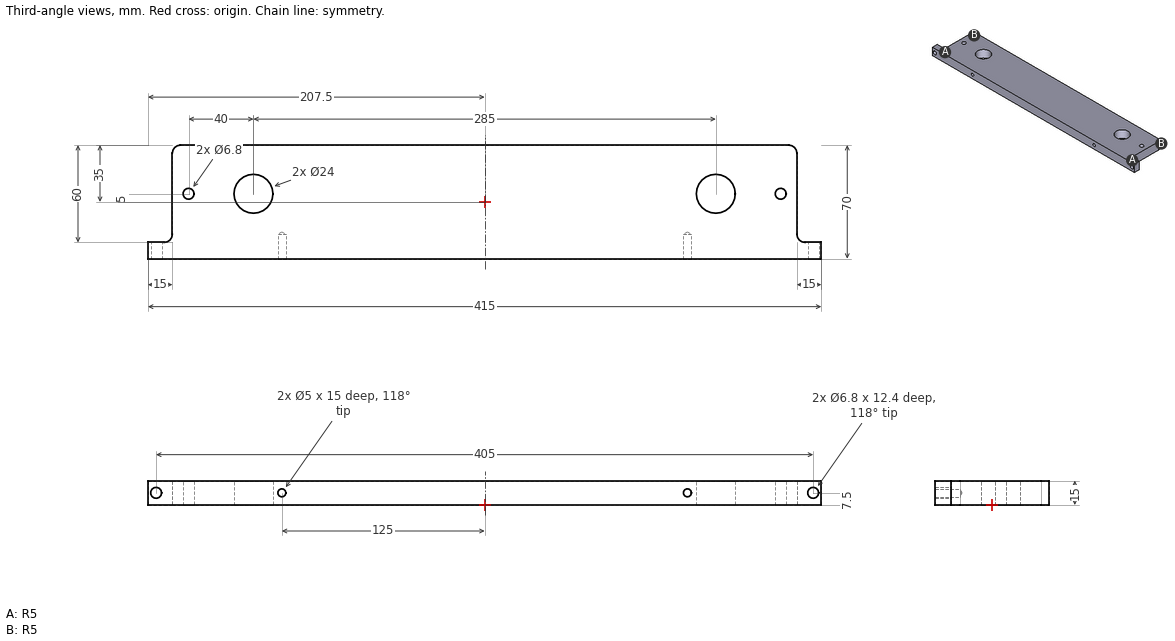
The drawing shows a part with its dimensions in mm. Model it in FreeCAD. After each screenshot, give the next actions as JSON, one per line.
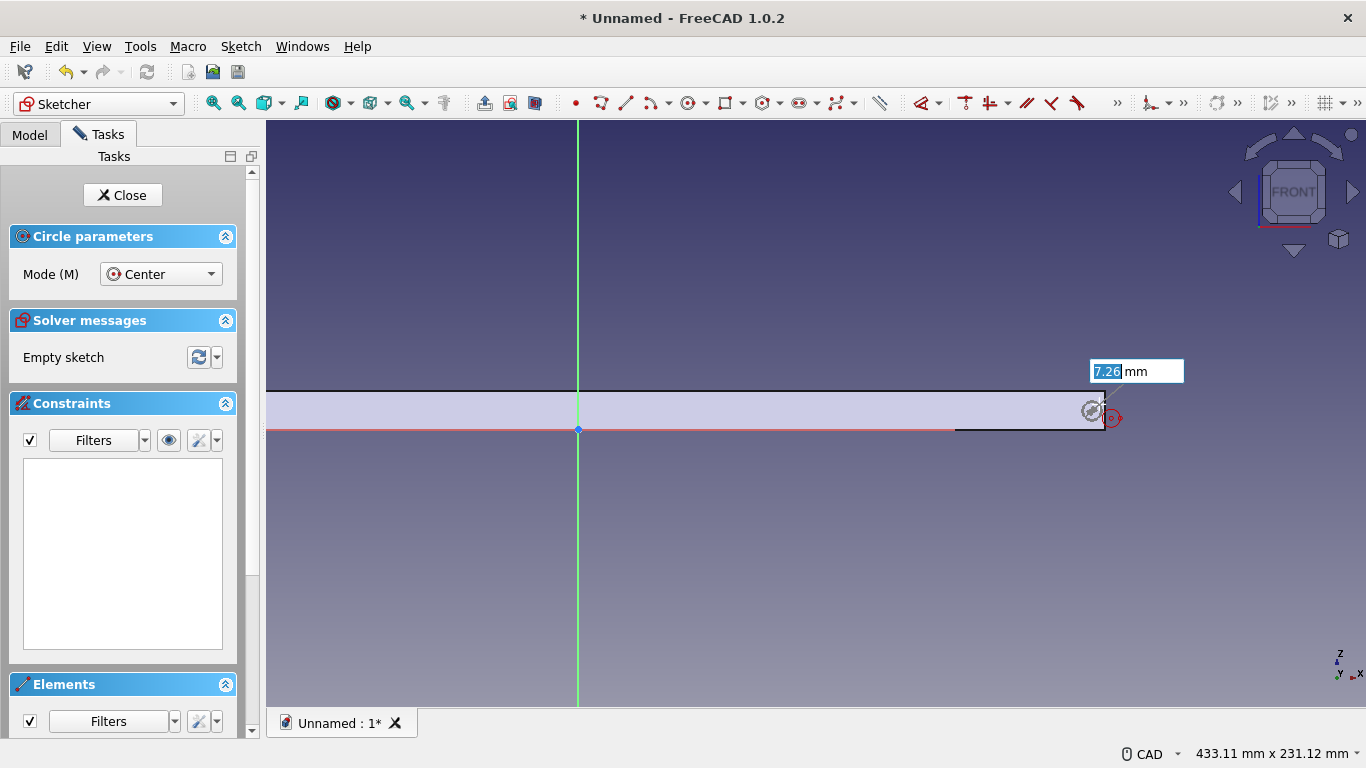
{"action": "type", "text": "6.8"}
{"action": "key", "text": "Return"}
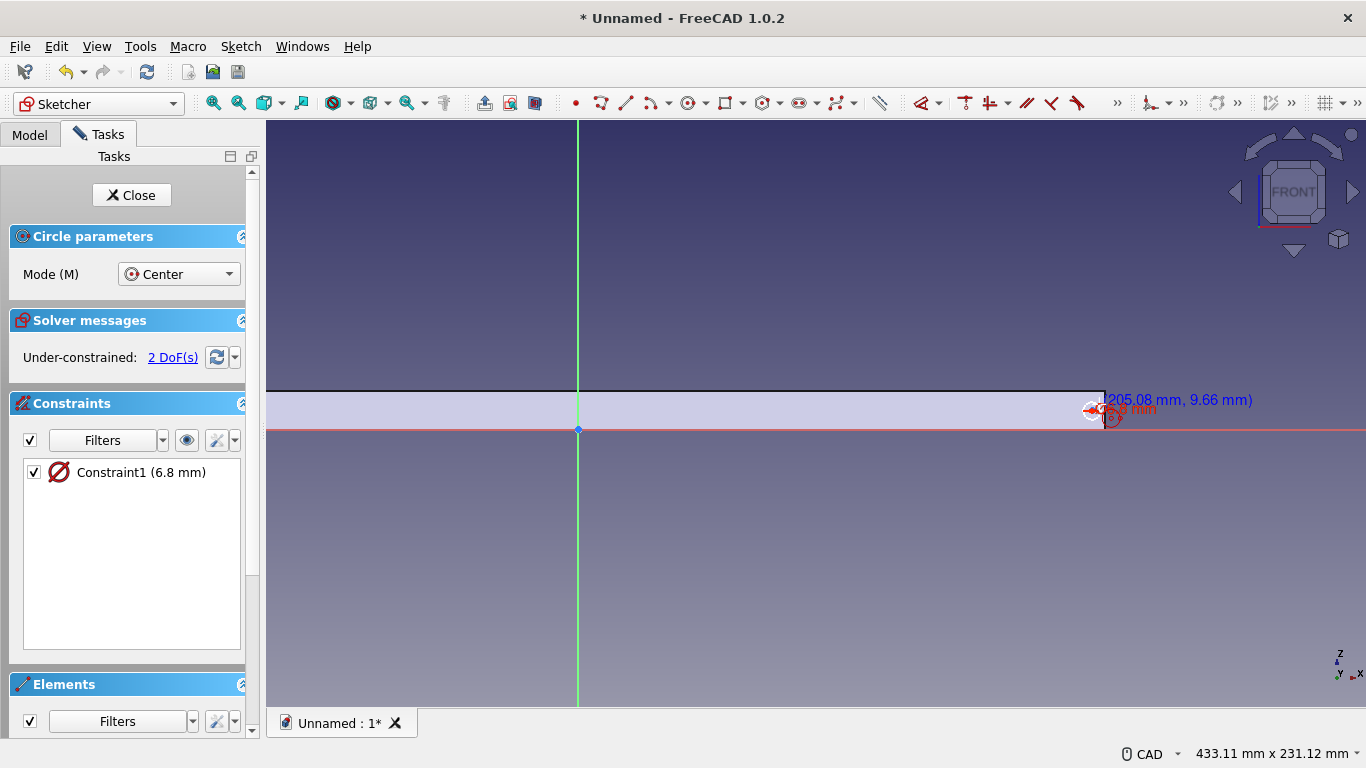
{"action": "scroll", "coordinate": [1092, 409], "scroll_direction": "down", "scroll_amount": 2}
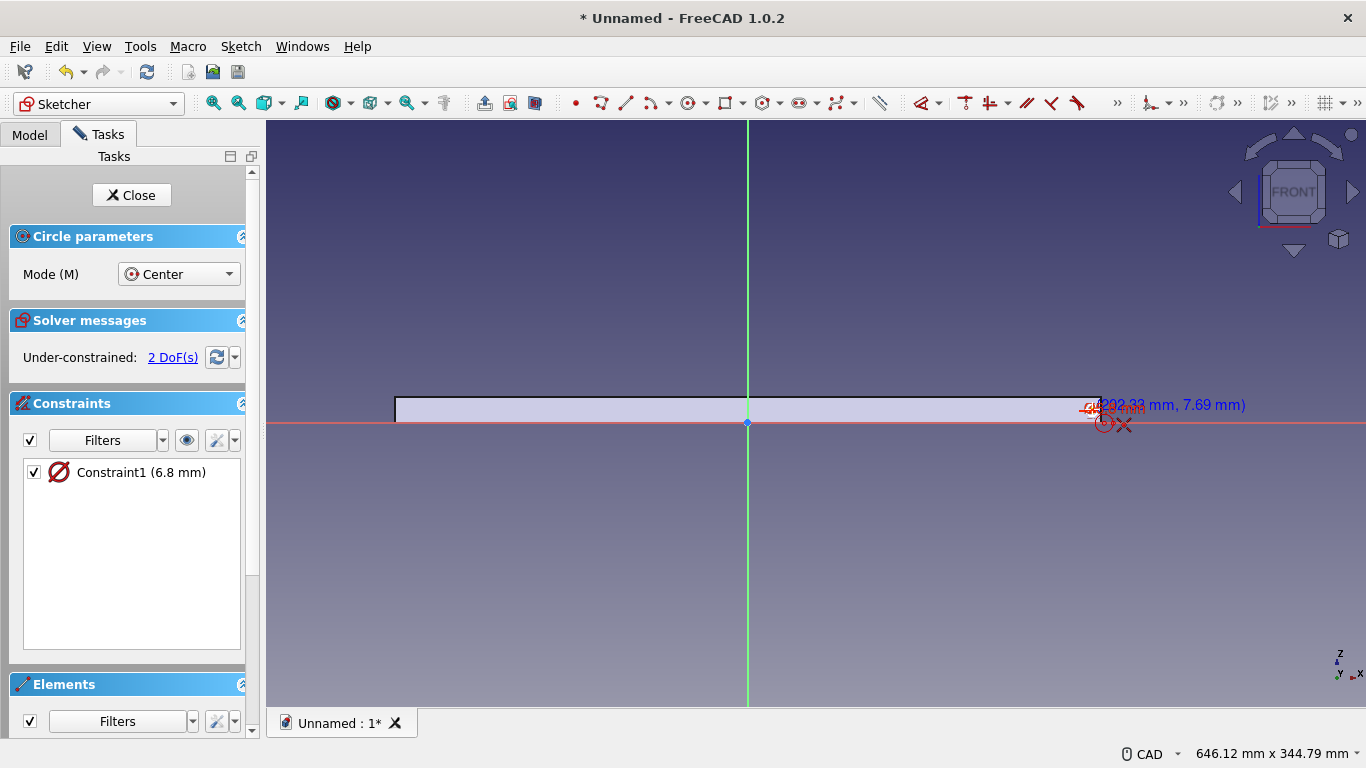
{"action": "scroll", "coordinate": [403, 410], "scroll_direction": "up", "scroll_amount": 7}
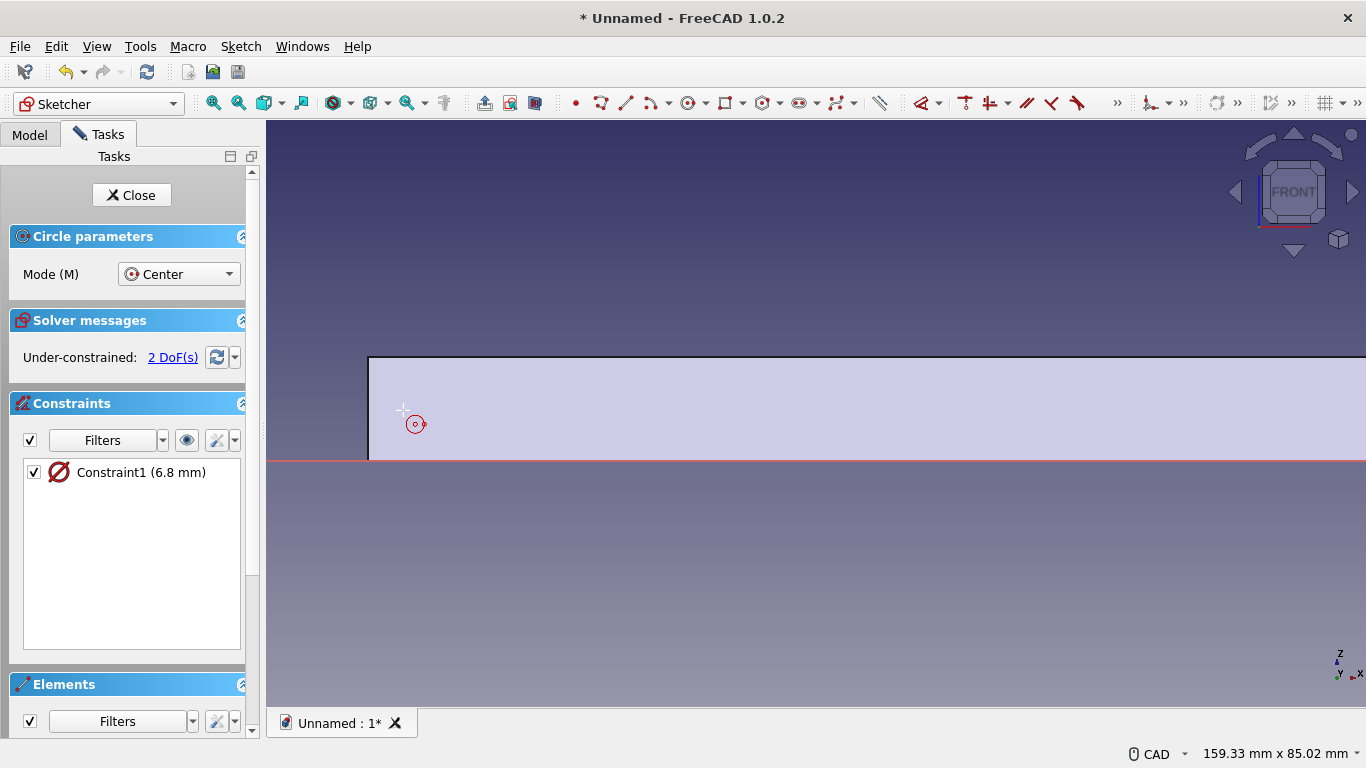
{"action": "scroll", "coordinate": [403, 410], "scroll_direction": "down", "scroll_amount": 7}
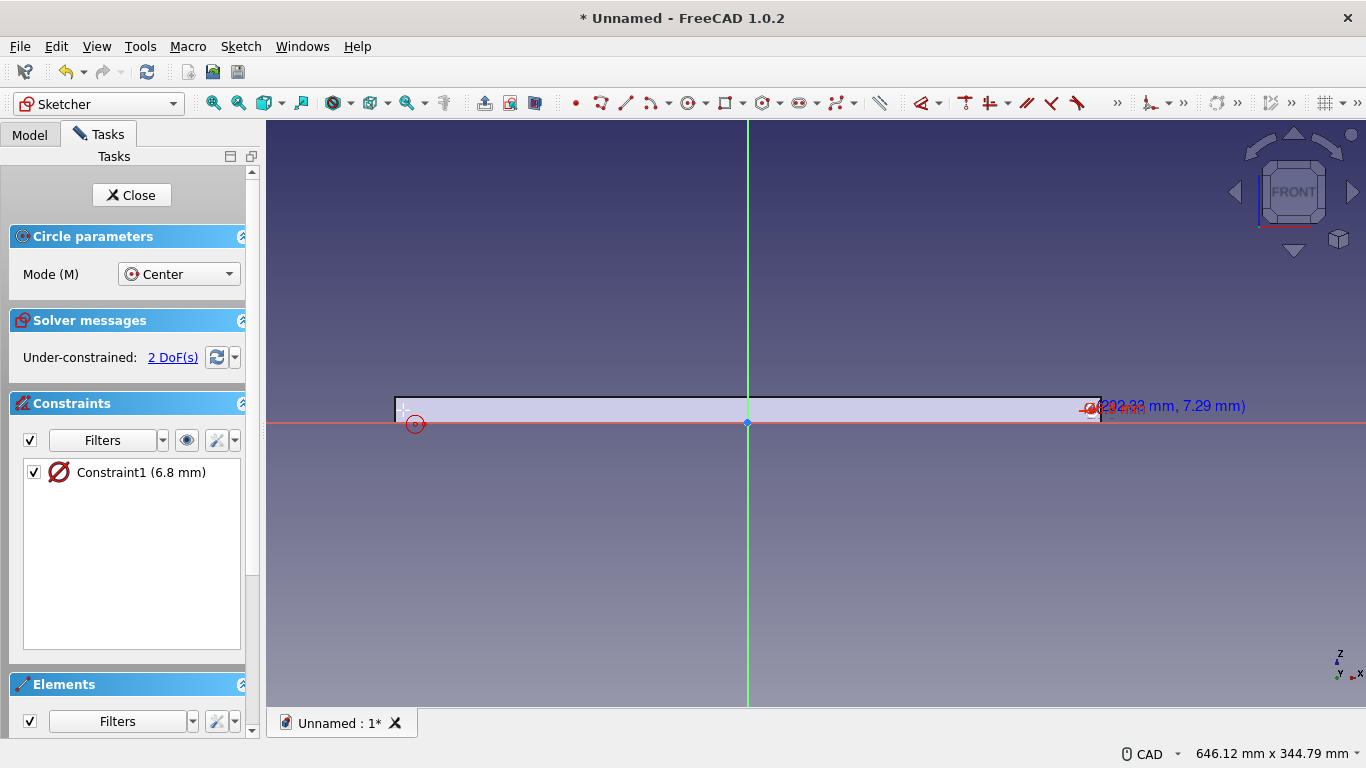
{"action": "scroll", "coordinate": [403, 410], "scroll_direction": "up", "scroll_amount": 2}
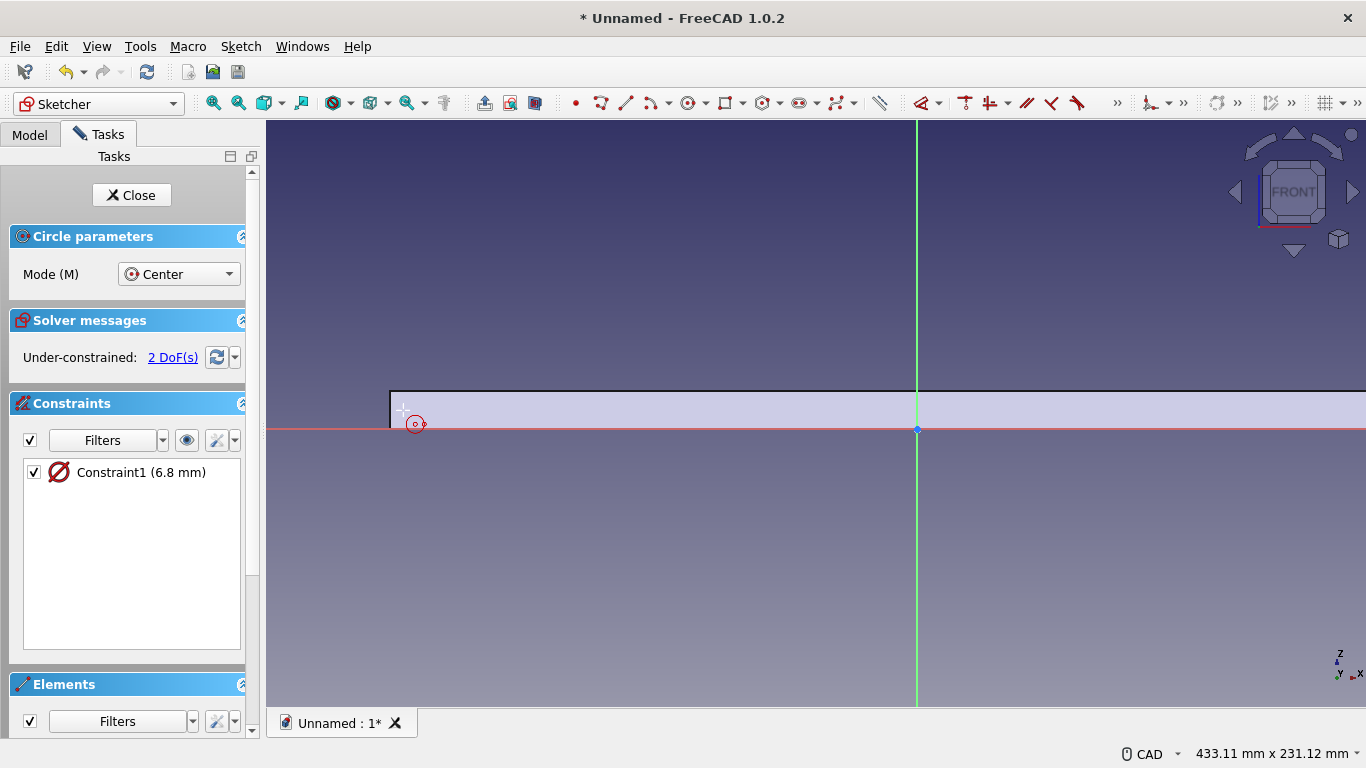
{"action": "left_click", "coordinate": [403, 410]}
{"action": "mouse_move", "coordinate": [409, 404]}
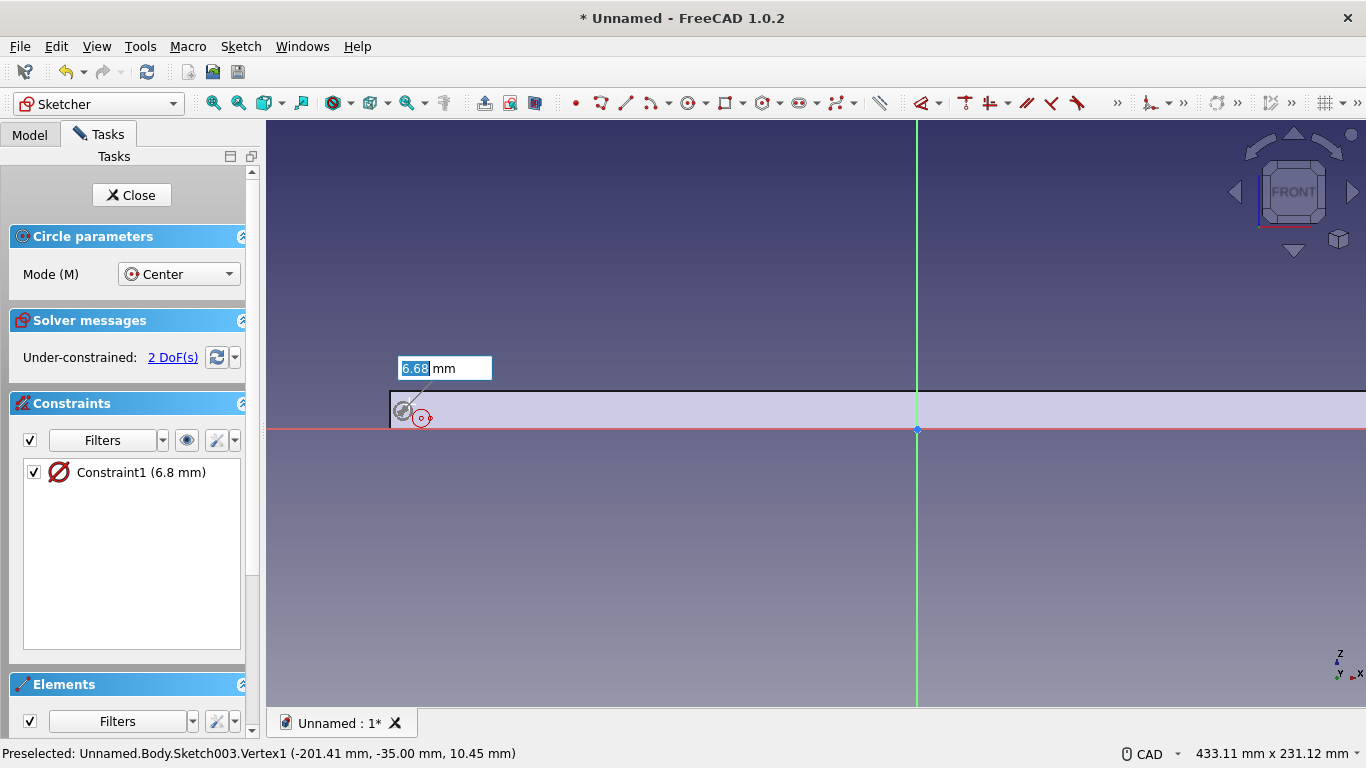
{"action": "type", "text": "6.8"}
{"action": "key", "text": "Return"}
{"action": "key", "text": "Escape"}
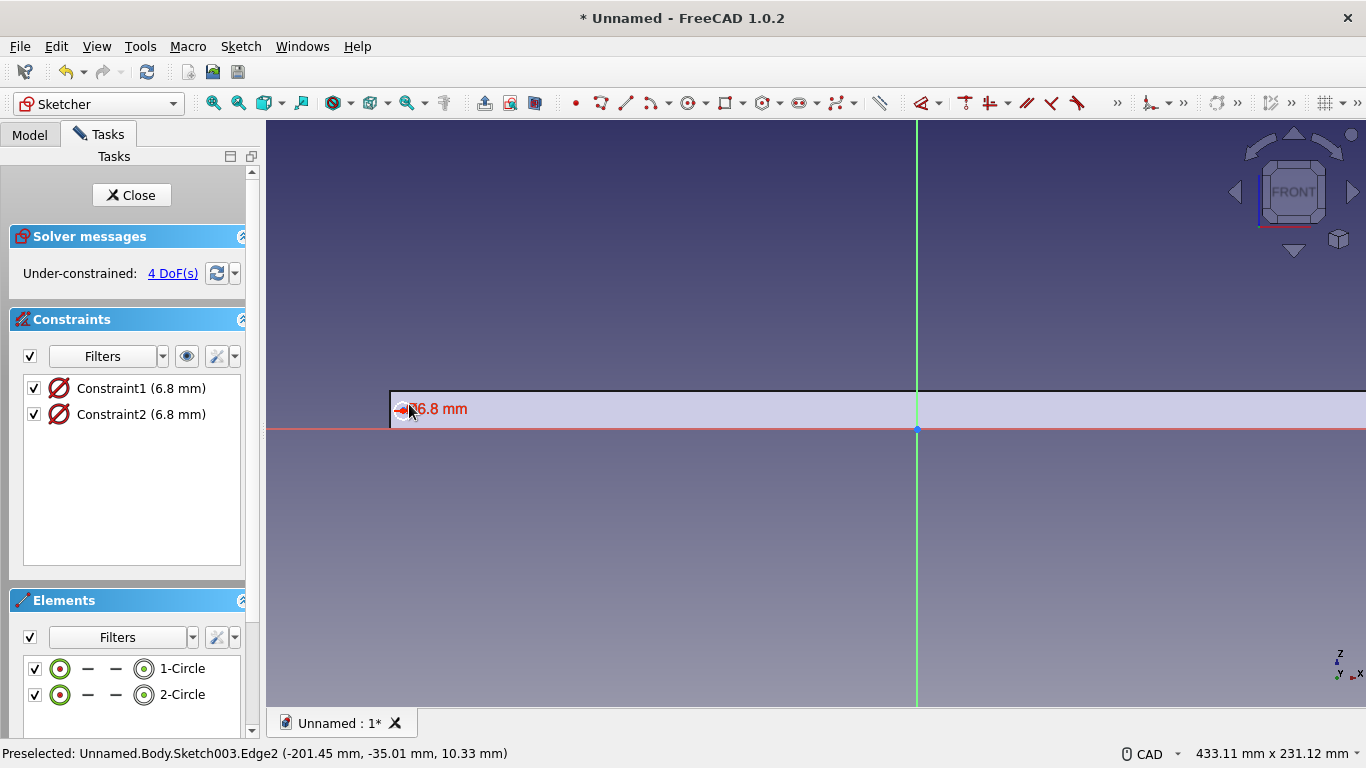
{"action": "scroll", "coordinate": [402, 410], "scroll_direction": "down", "scroll_amount": 2}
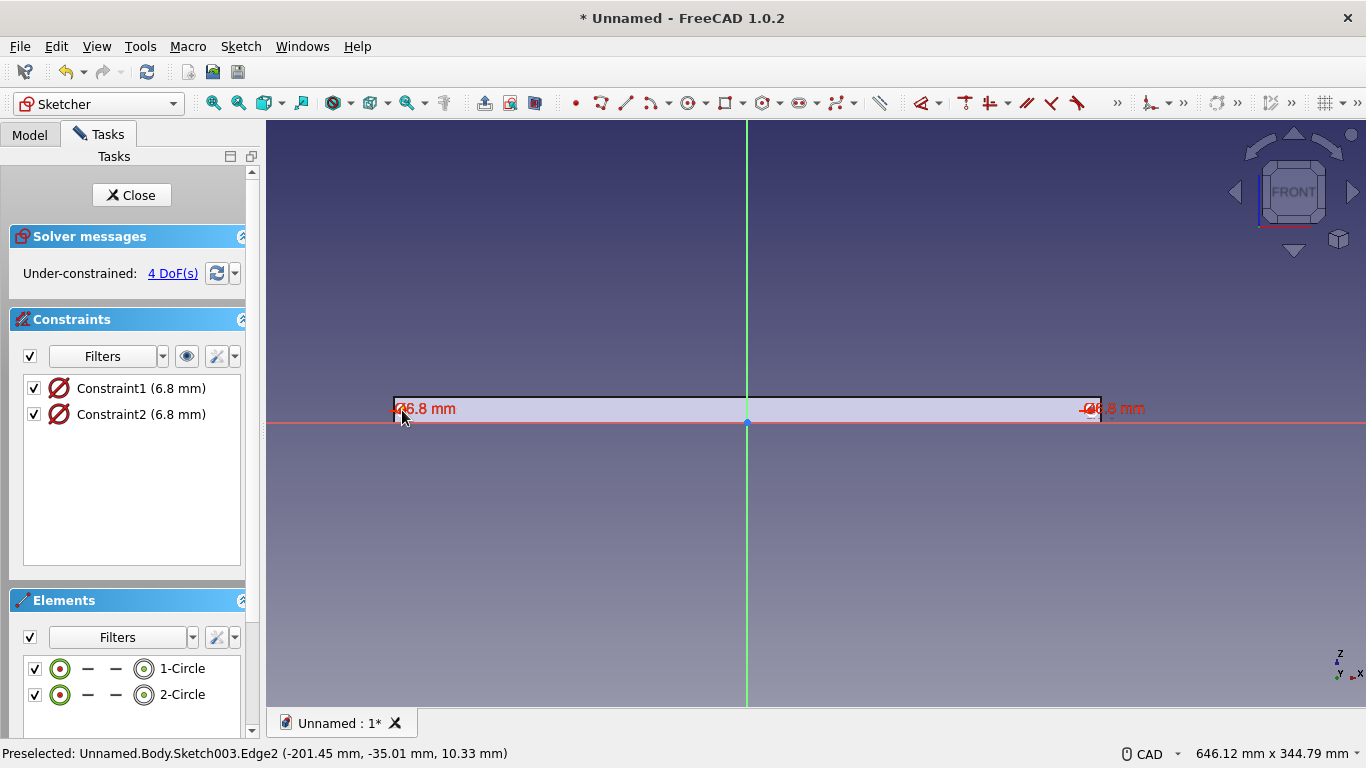
{"action": "left_click", "coordinate": [1092, 411]}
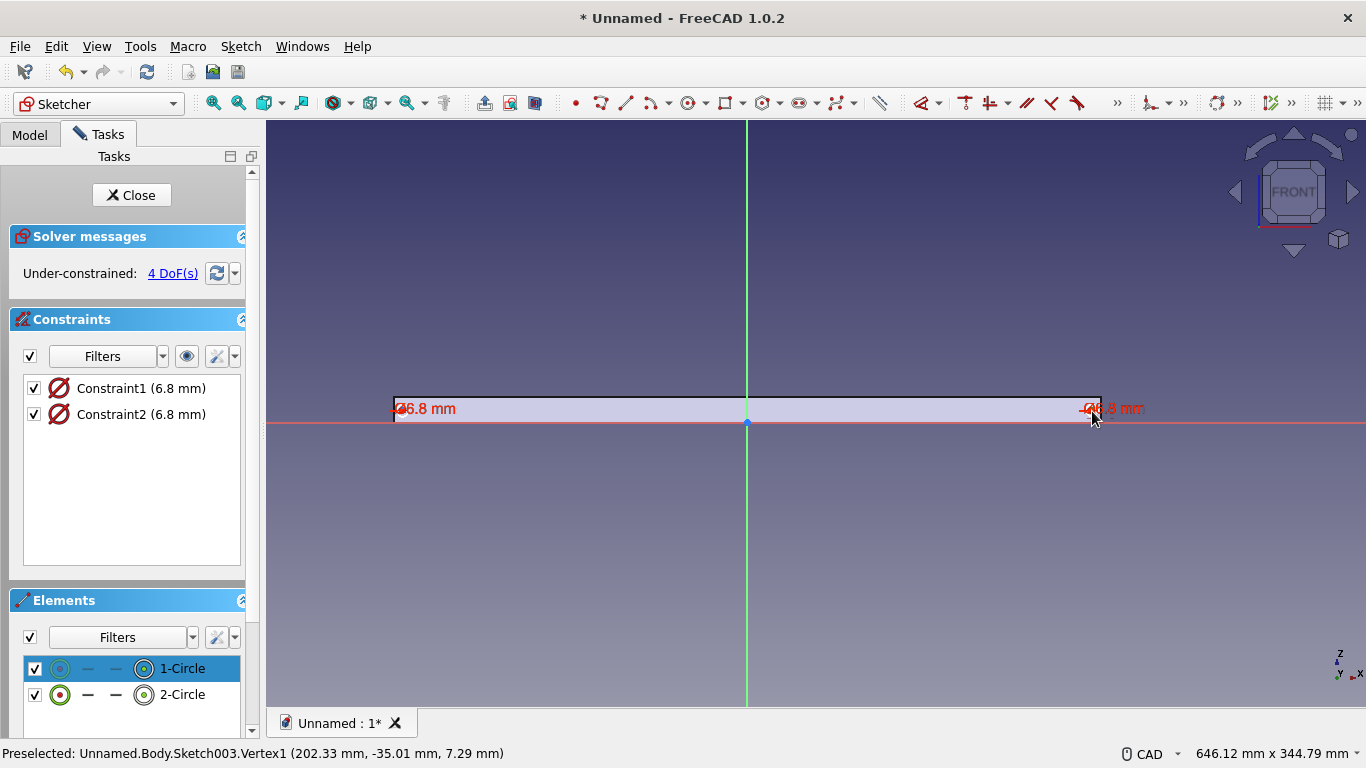
{"action": "left_click", "coordinate": [403, 411]}